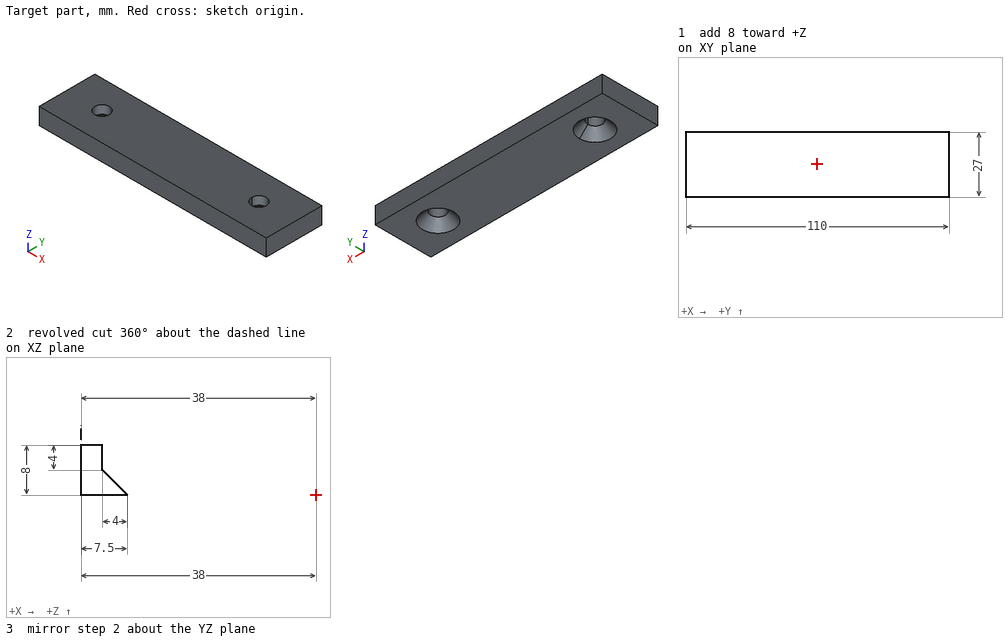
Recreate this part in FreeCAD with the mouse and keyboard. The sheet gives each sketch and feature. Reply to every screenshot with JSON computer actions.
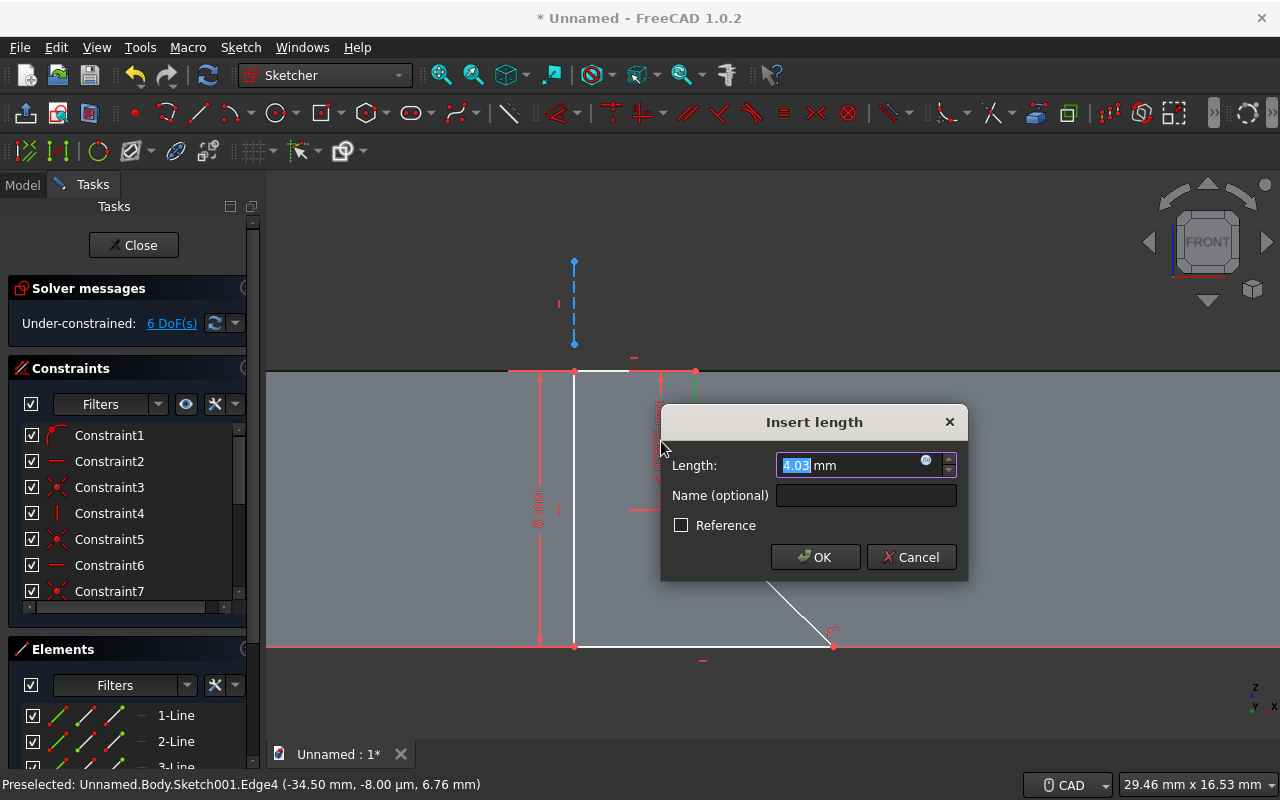
{"action": "type", "text": "4"}
{"action": "key", "text": "Return"}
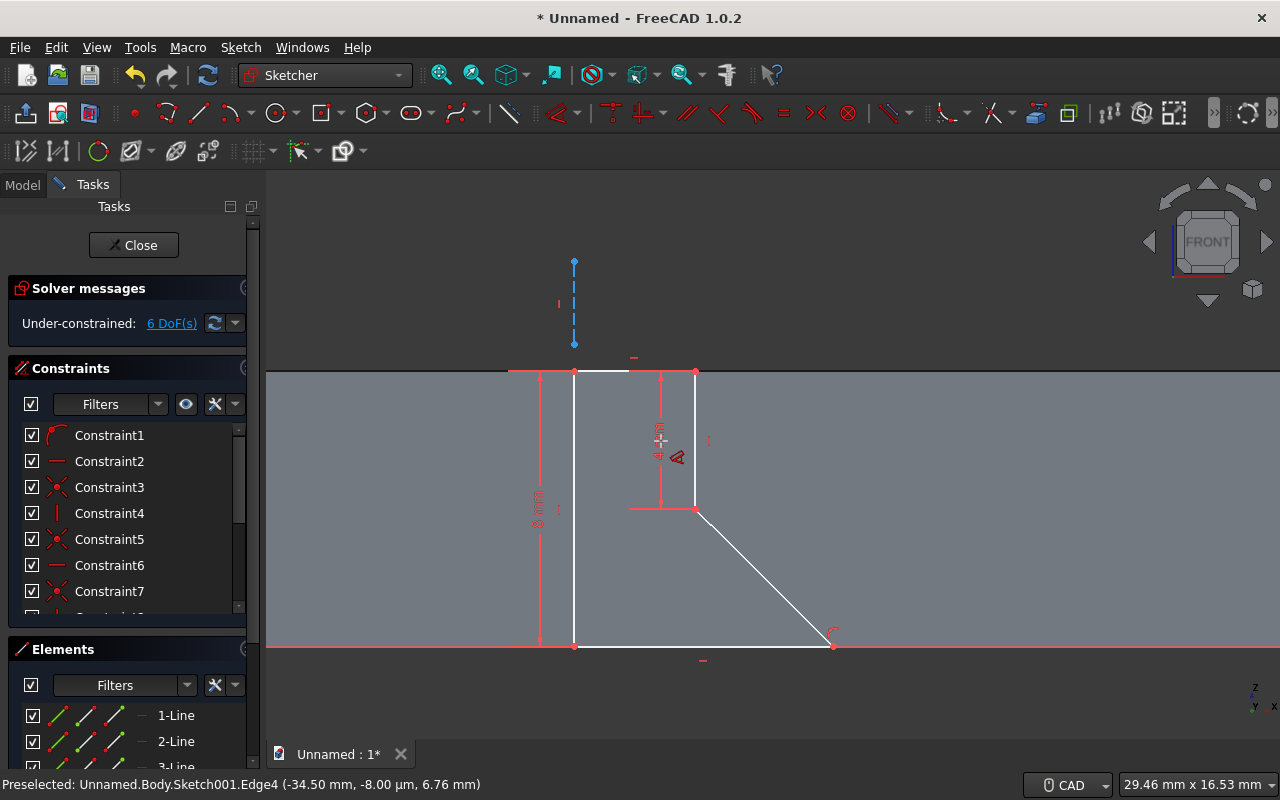
{"action": "left_click", "coordinate": [736, 550]}
{"action": "left_click", "coordinate": [764, 681]}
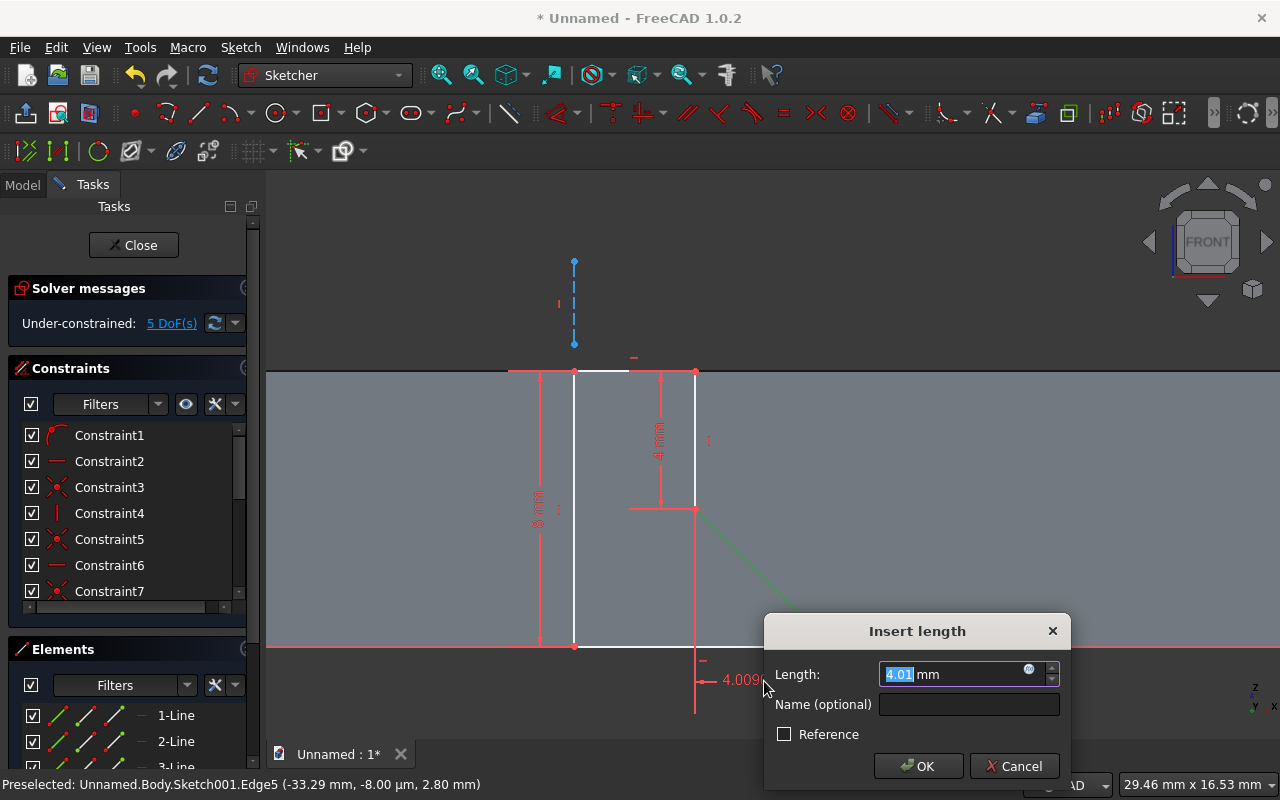
{"action": "type", "text": "4"}
{"action": "key", "text": "Return"}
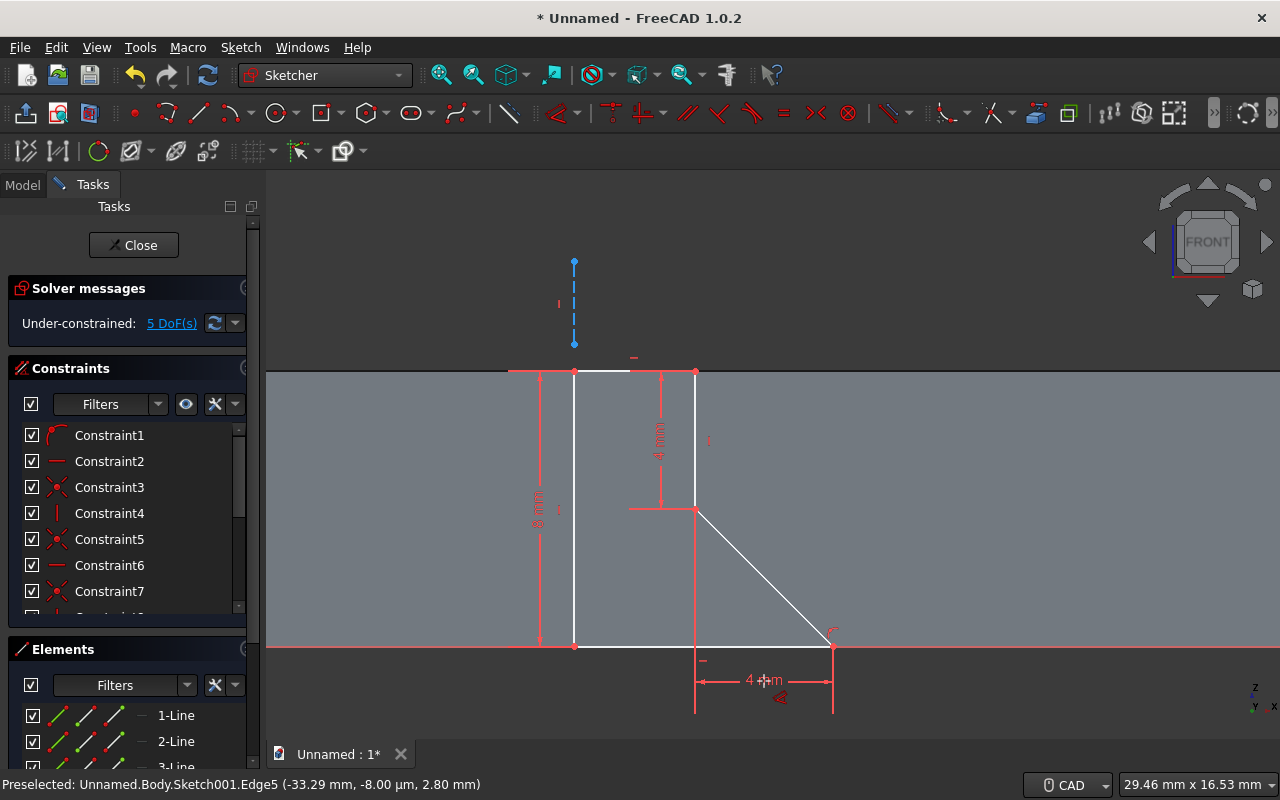
{"action": "left_click", "coordinate": [755, 647]}
{"action": "left_click", "coordinate": [644, 681]}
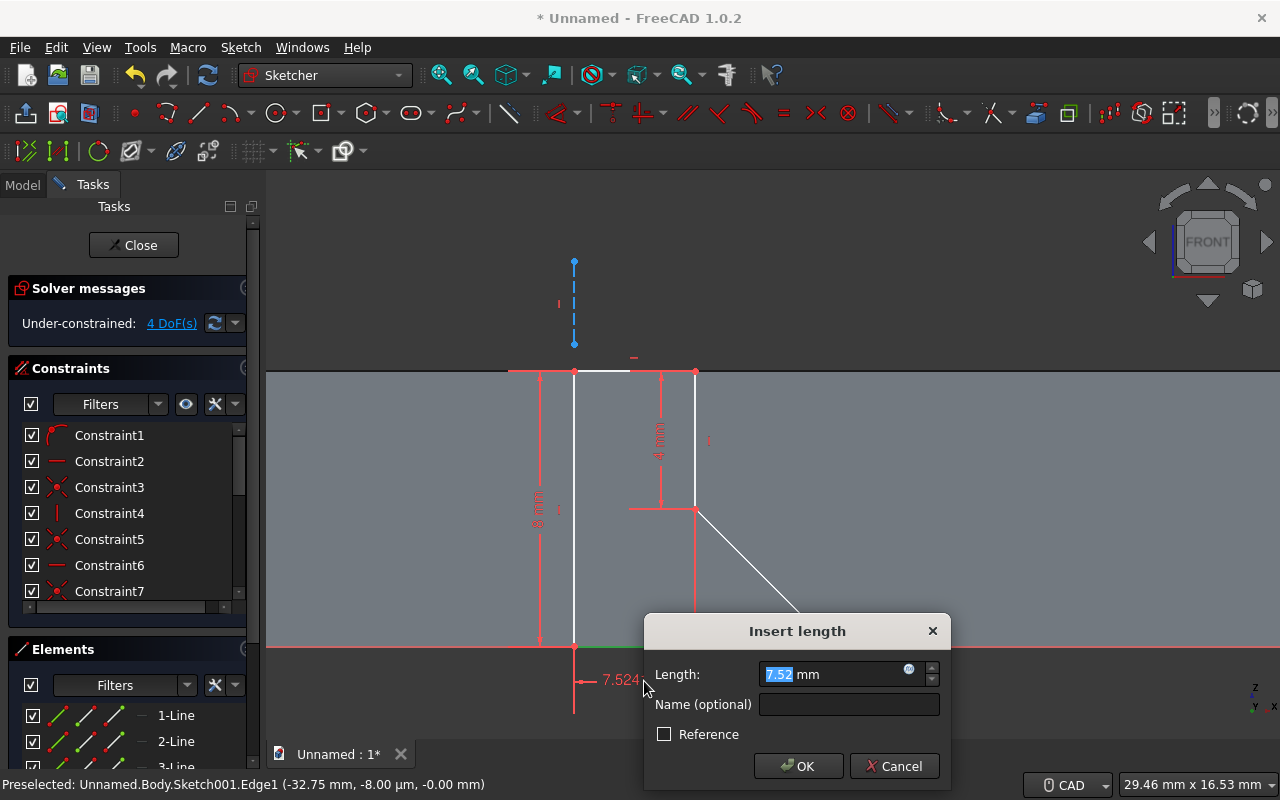
{"action": "type", "text": "7.5"}
{"action": "key", "text": "Return"}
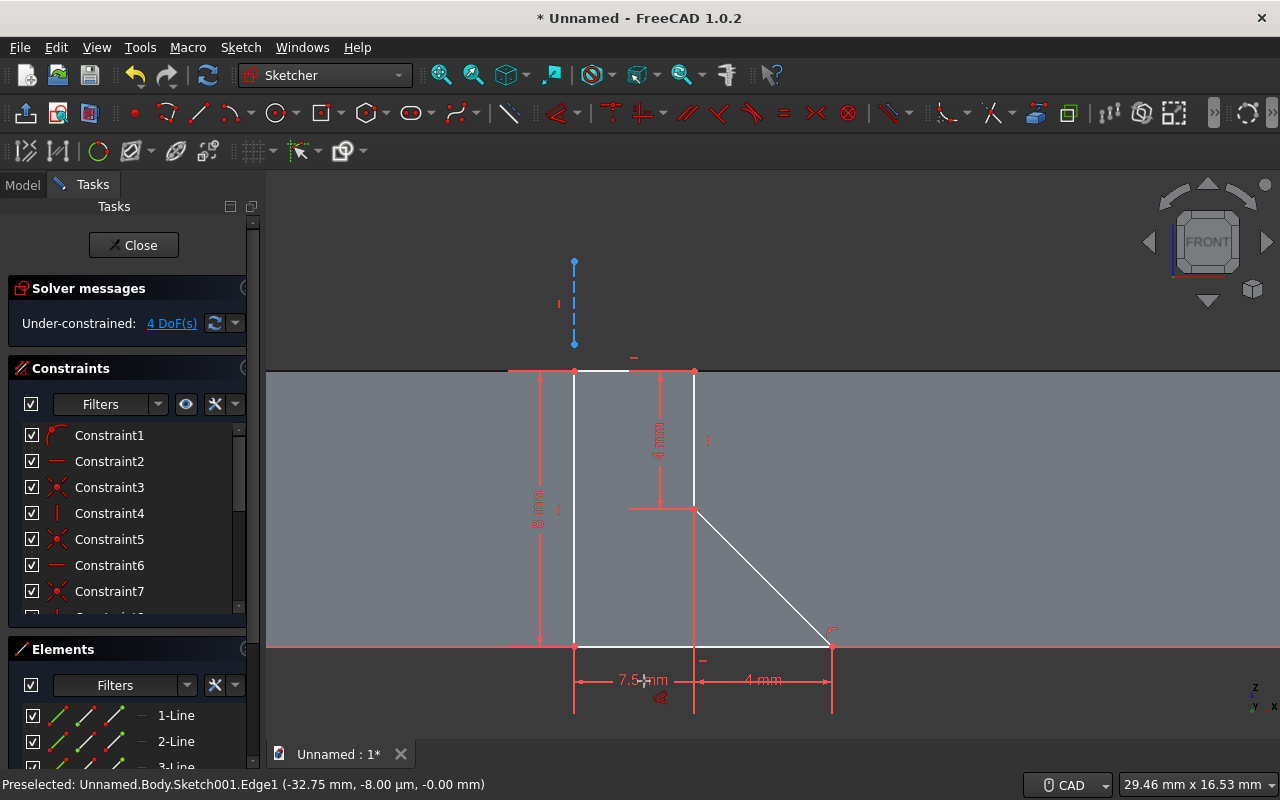
{"action": "left_click", "coordinate": [574, 647]}
{"action": "left_click", "coordinate": [844, 681]}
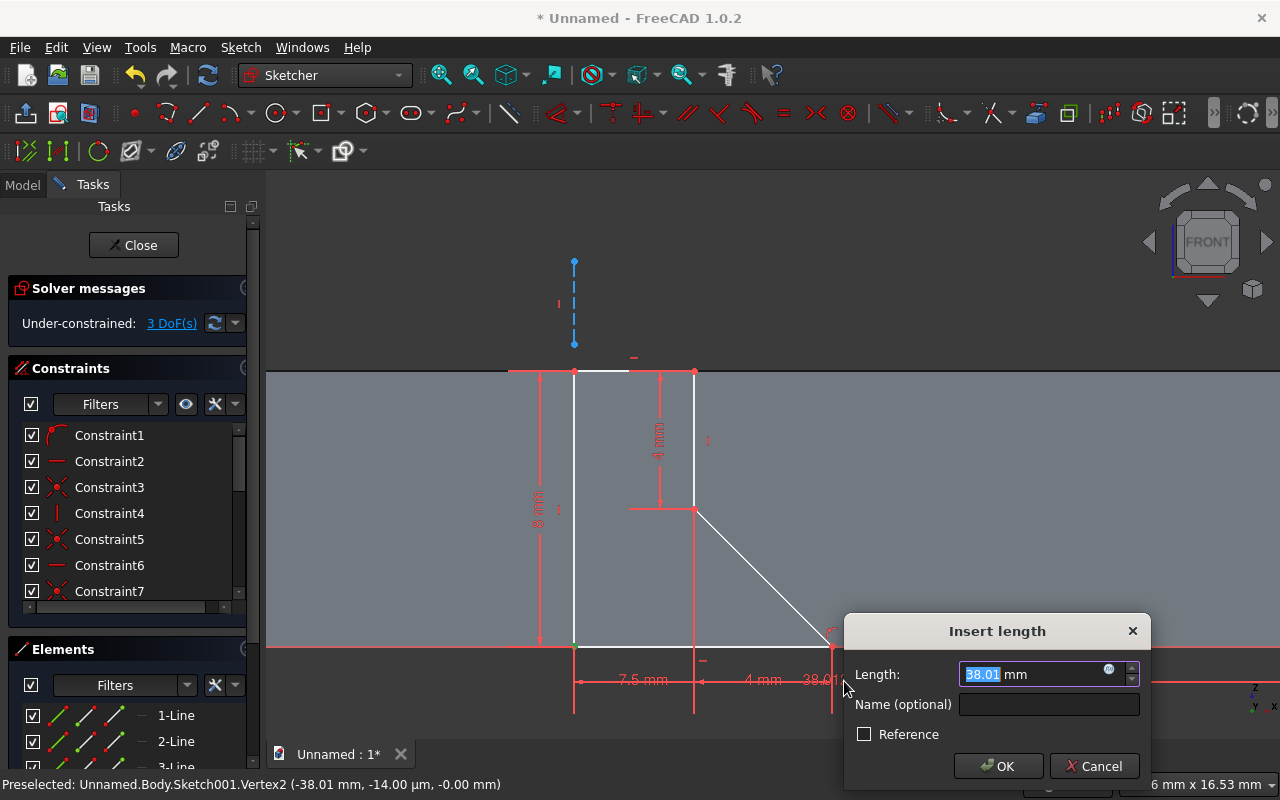
{"action": "type", "text": "38"}
{"action": "key", "text": "Return"}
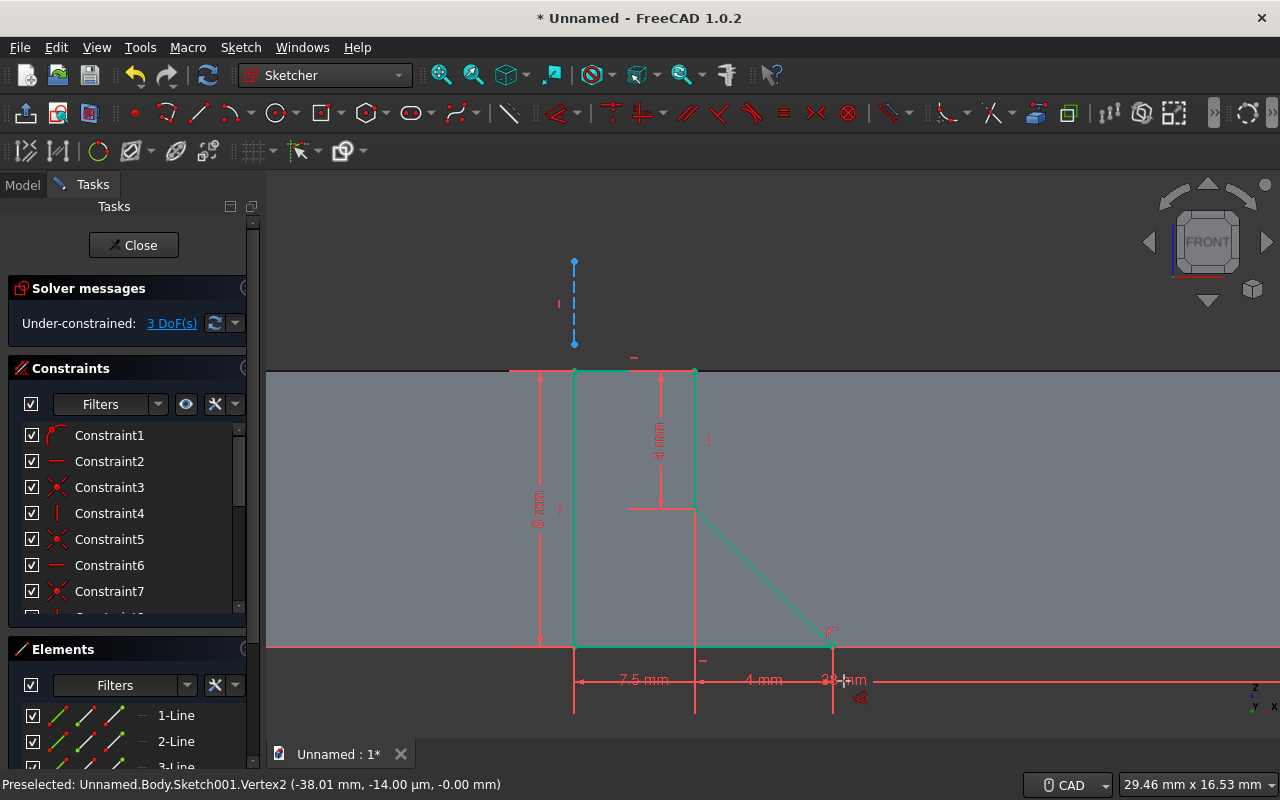
{"action": "left_click", "coordinate": [574, 345]}
{"action": "left_click", "coordinate": [969, 681]}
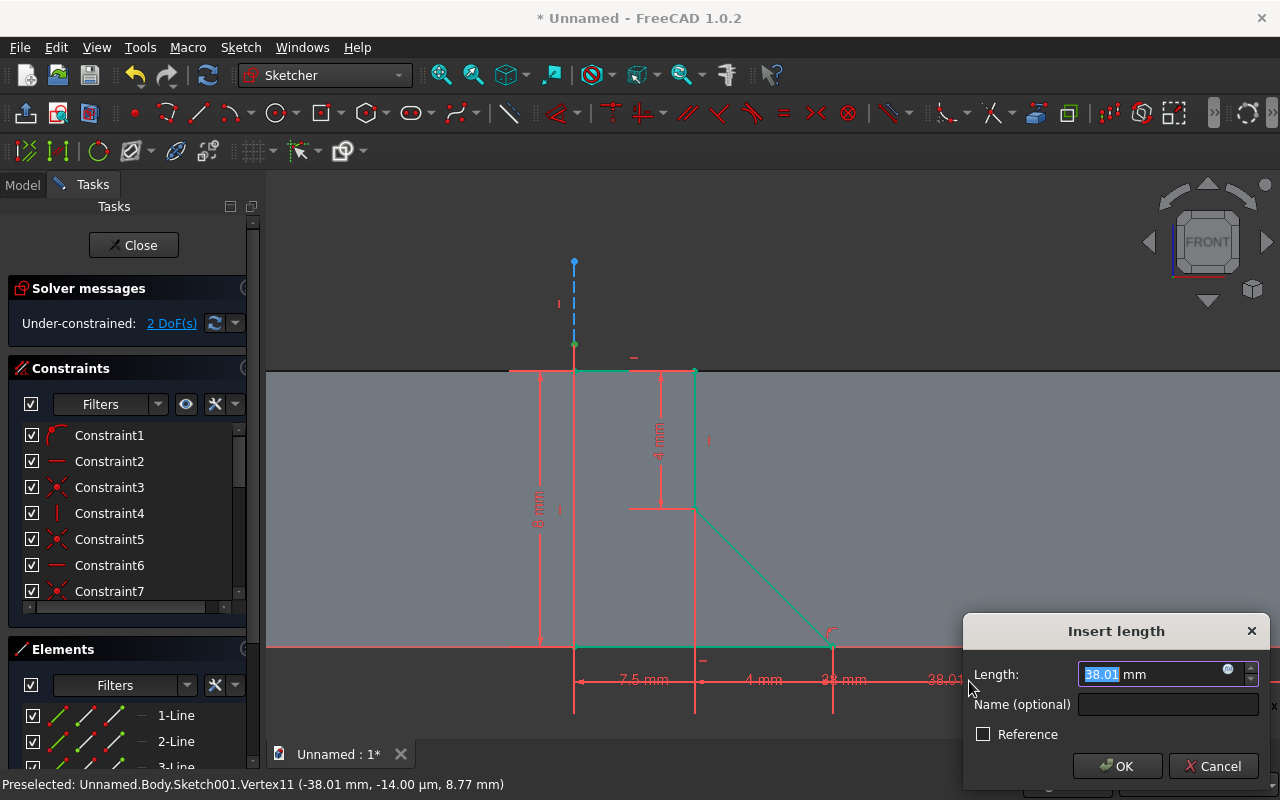
{"action": "type", "text": "38"}
{"action": "key", "text": "Return"}
{"action": "key", "text": "Escape"}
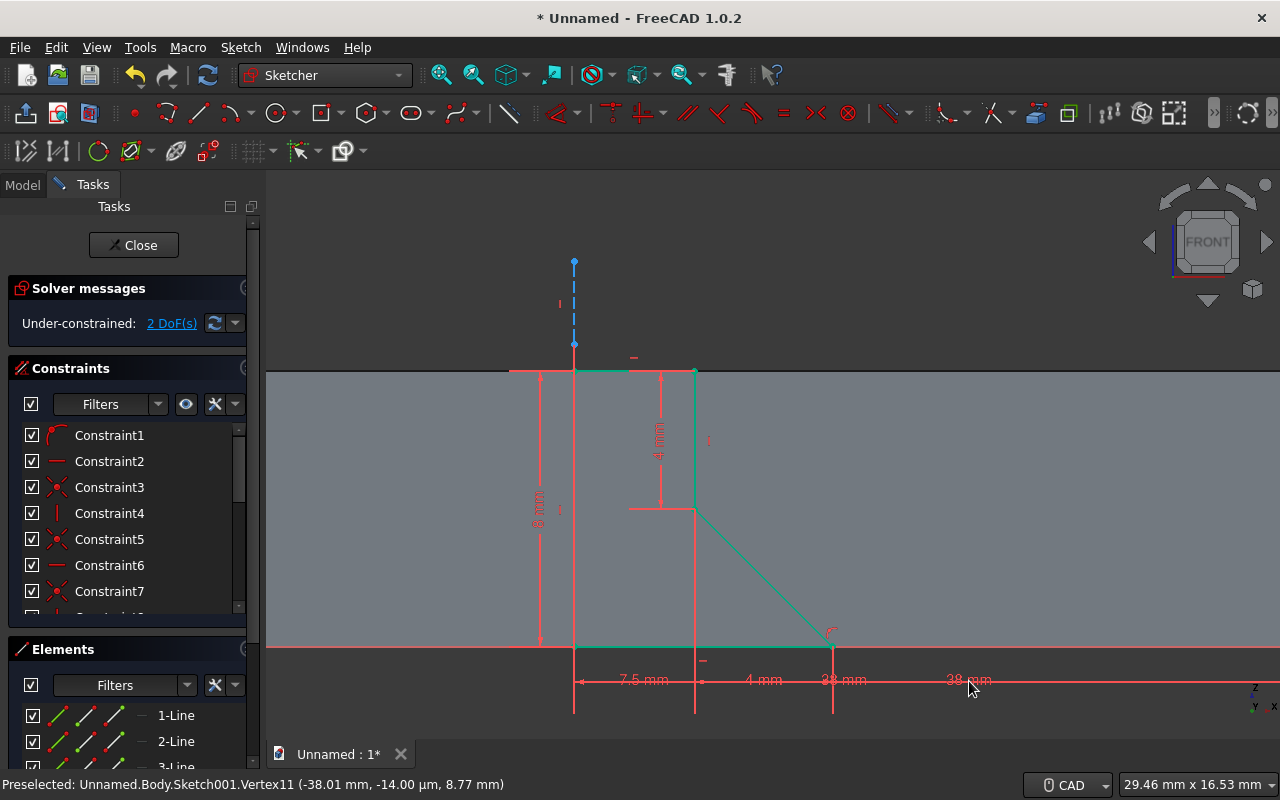
{"action": "left_click", "coordinate": [134, 245]}